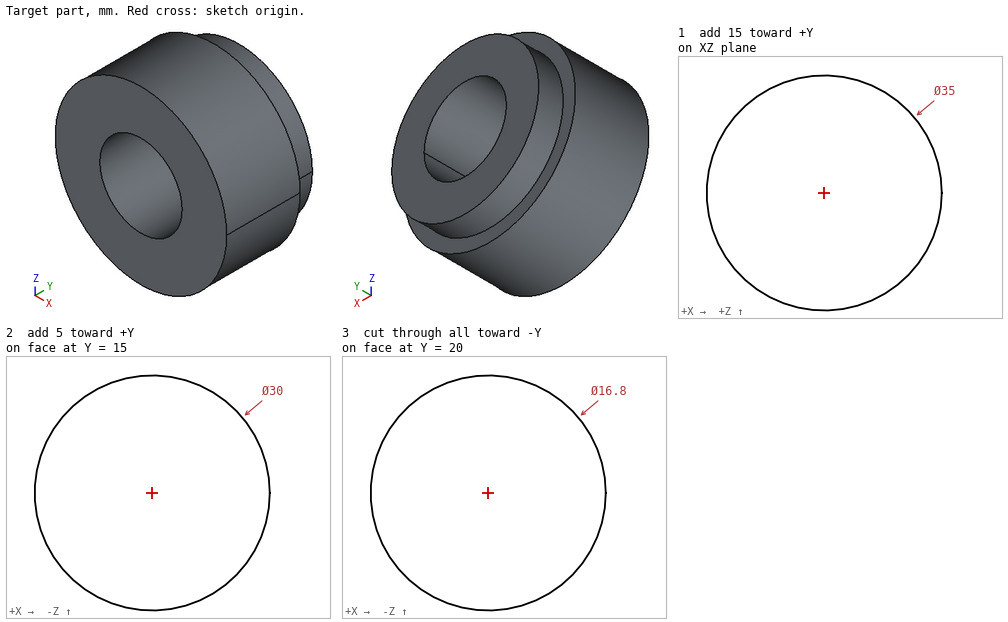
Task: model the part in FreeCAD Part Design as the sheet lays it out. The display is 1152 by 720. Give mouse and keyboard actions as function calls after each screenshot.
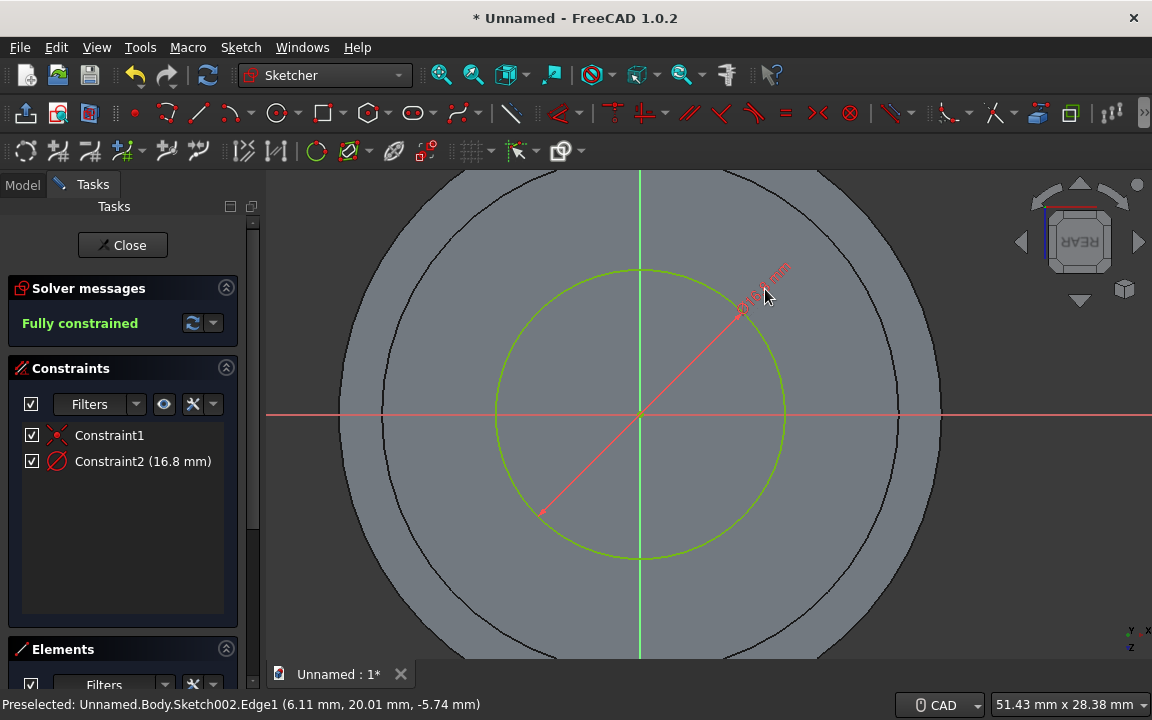
click(123, 245)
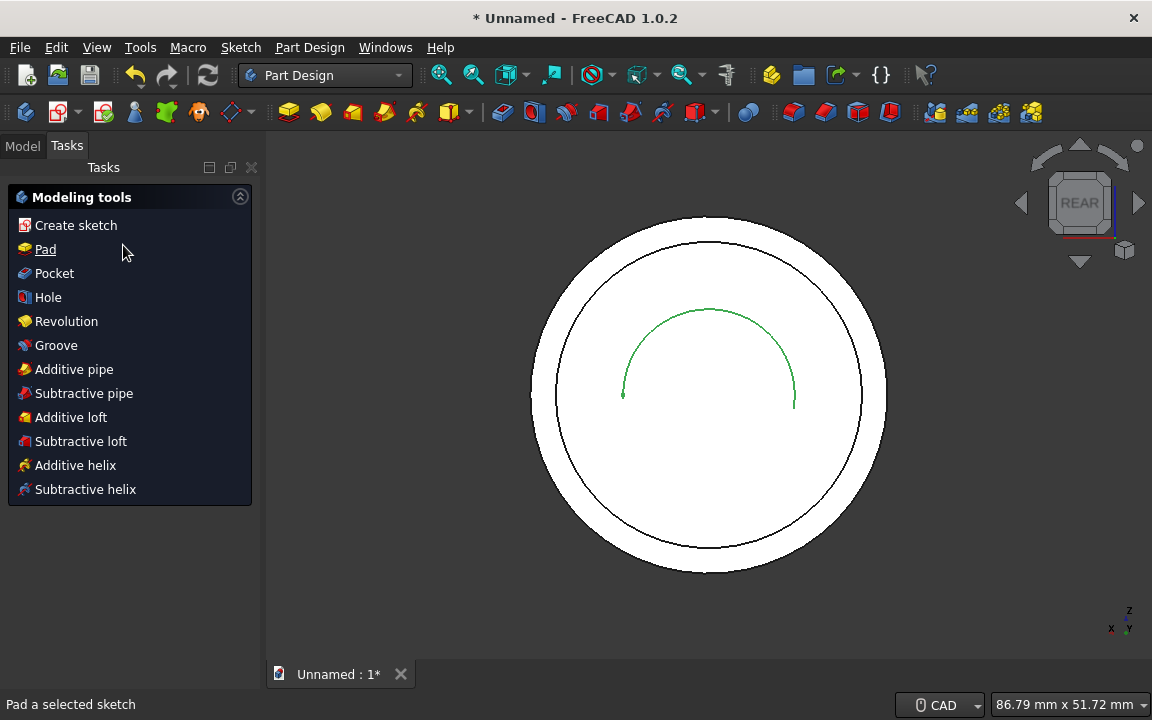
click(504, 112)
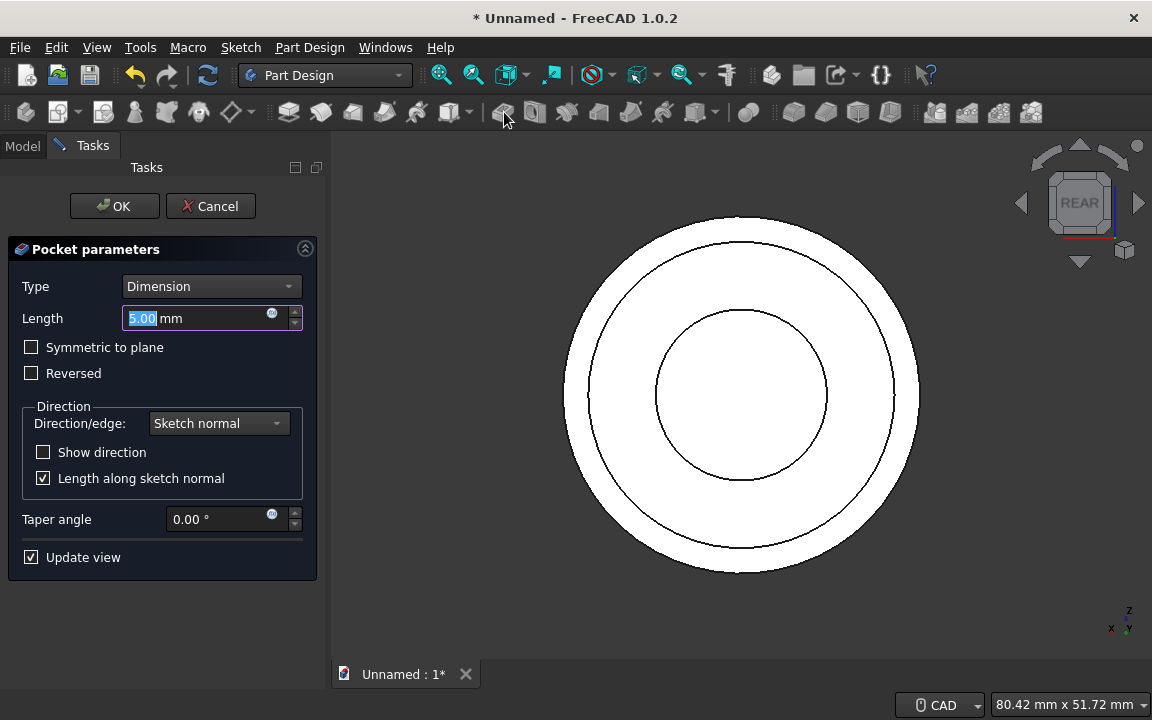
click(212, 286)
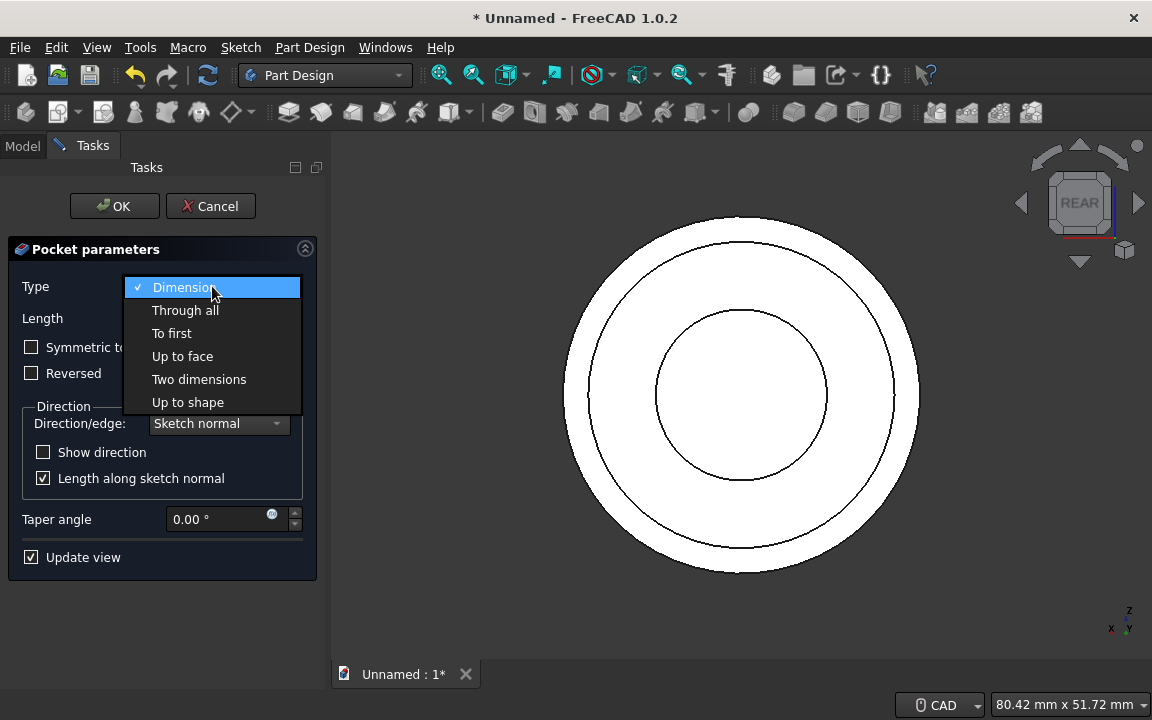
click(212, 310)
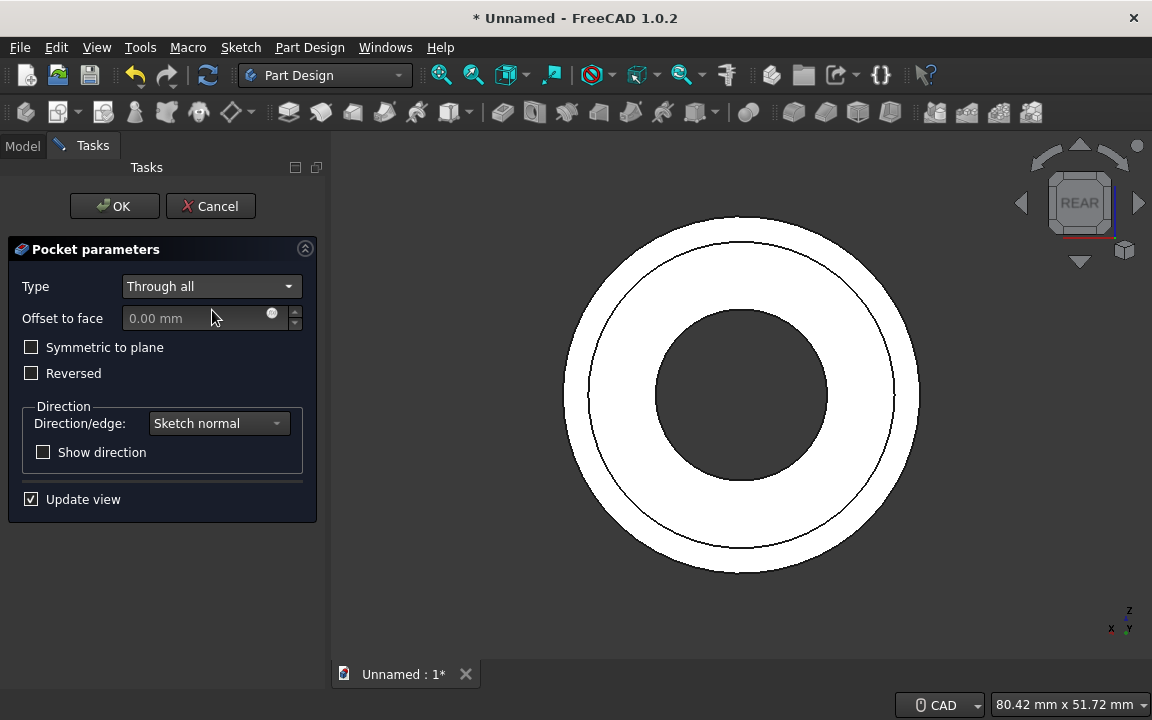
click(115, 206)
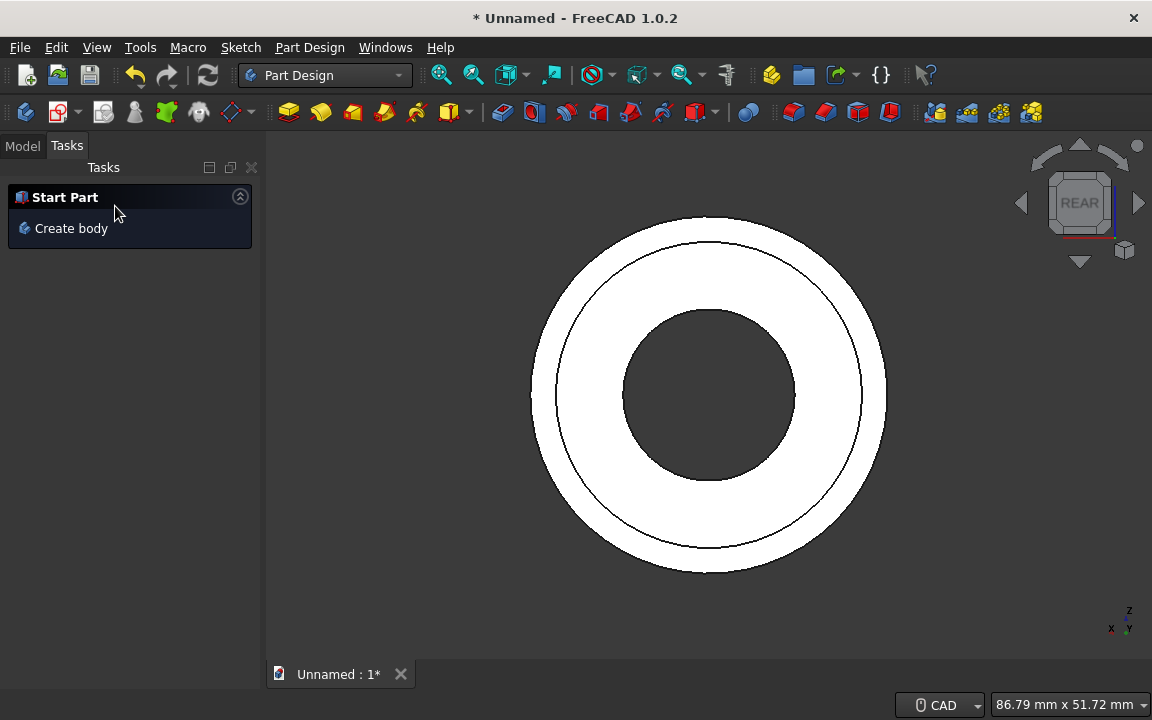
key(0)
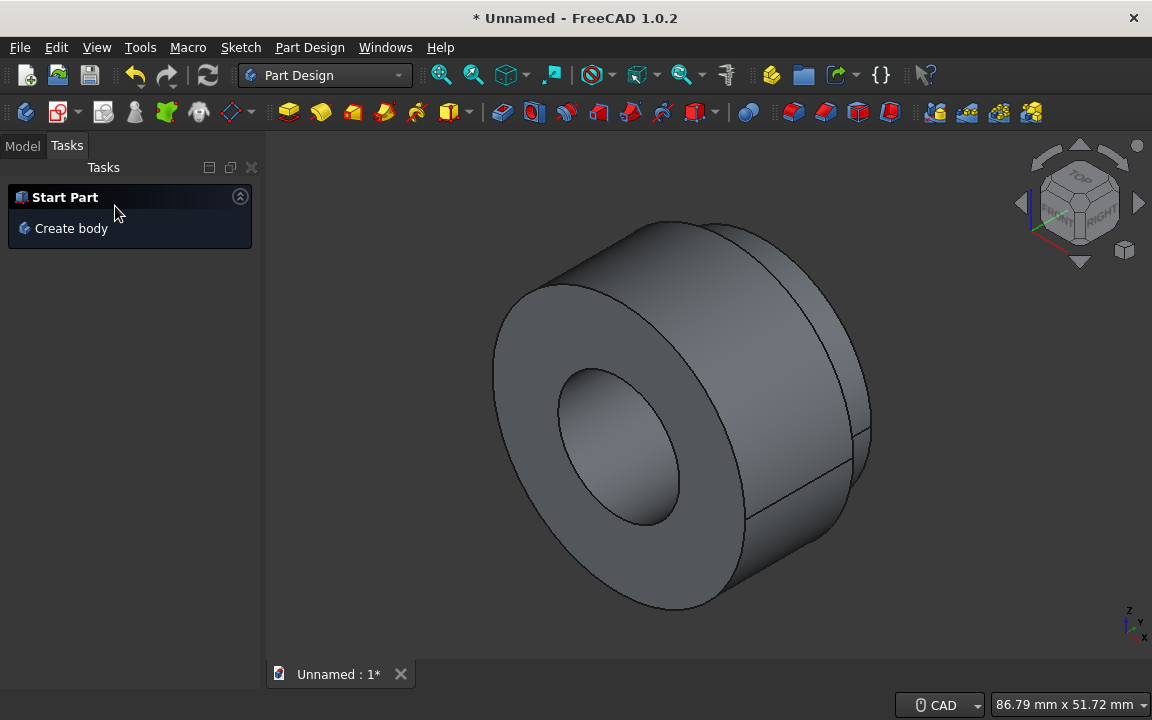
click(442, 76)